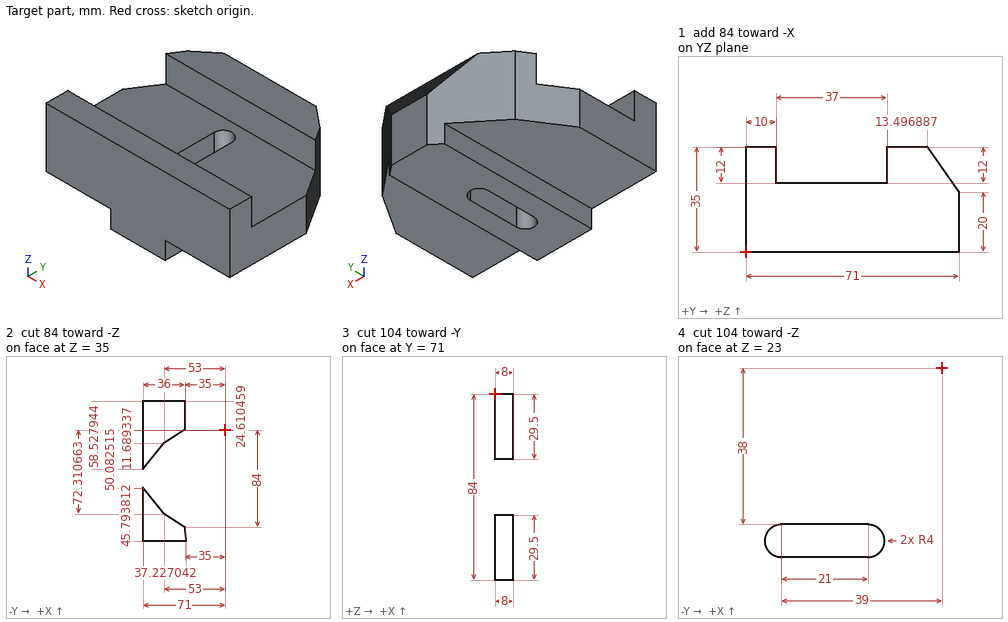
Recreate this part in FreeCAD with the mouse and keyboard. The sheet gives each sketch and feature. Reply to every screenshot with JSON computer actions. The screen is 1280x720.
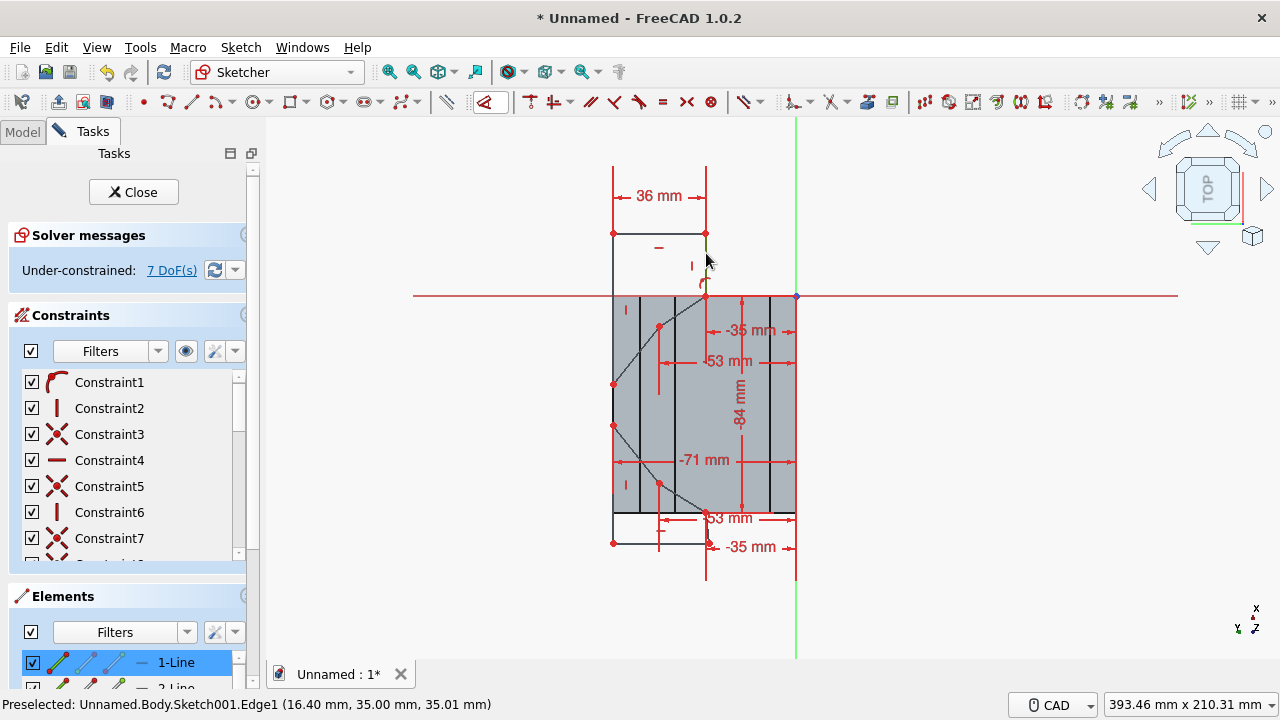
{"action": "left_click", "coordinate": [502, 102]}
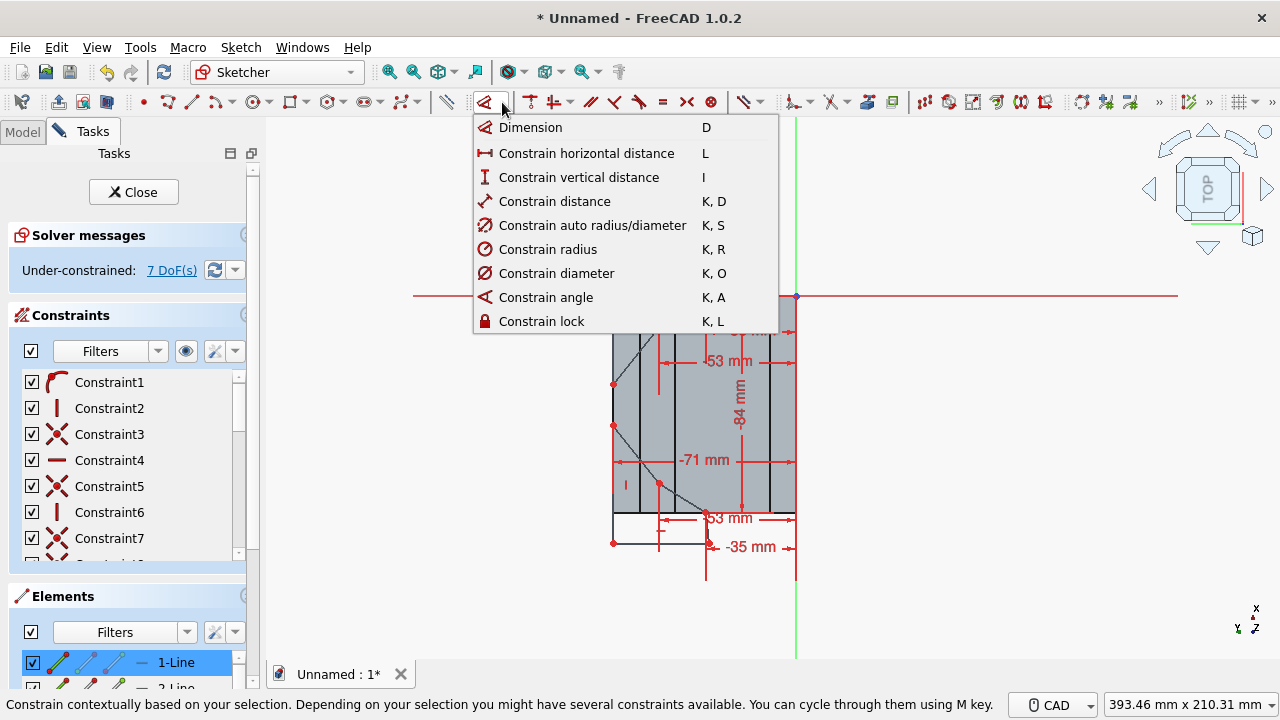
{"action": "left_click", "coordinate": [626, 177]}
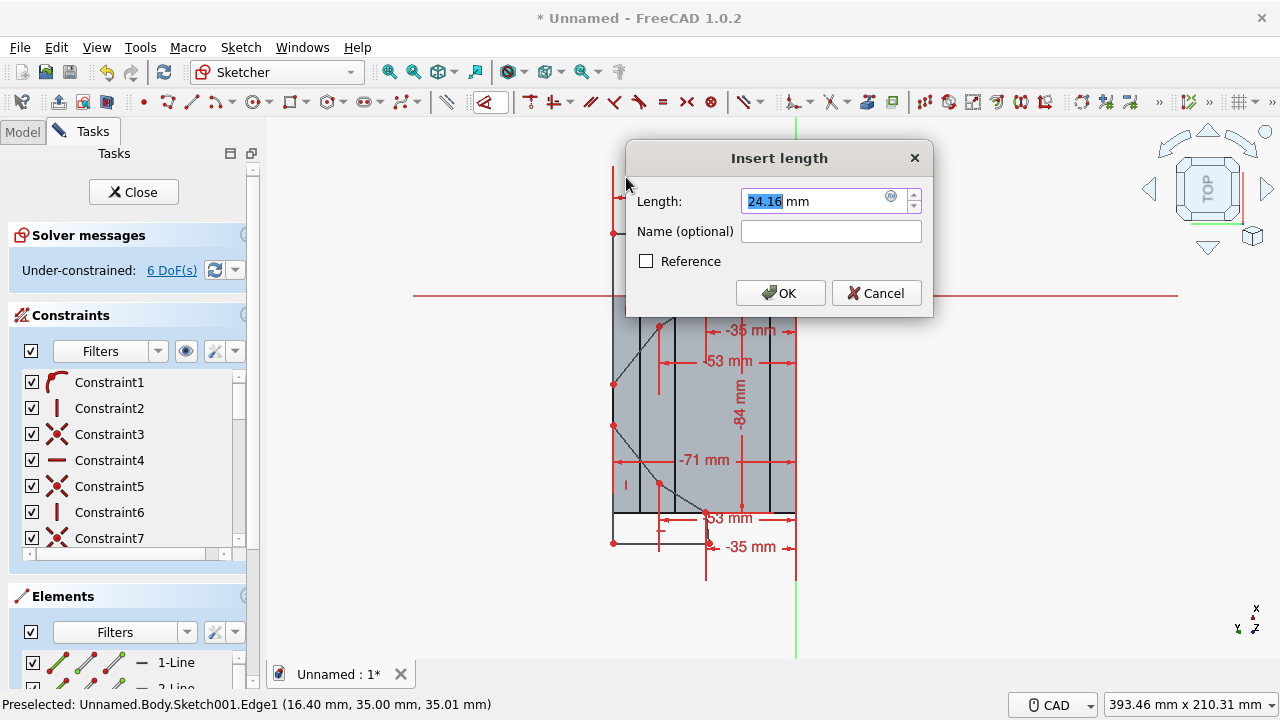
{"action": "type", "text": "24.610459"}
{"action": "key", "text": "Return"}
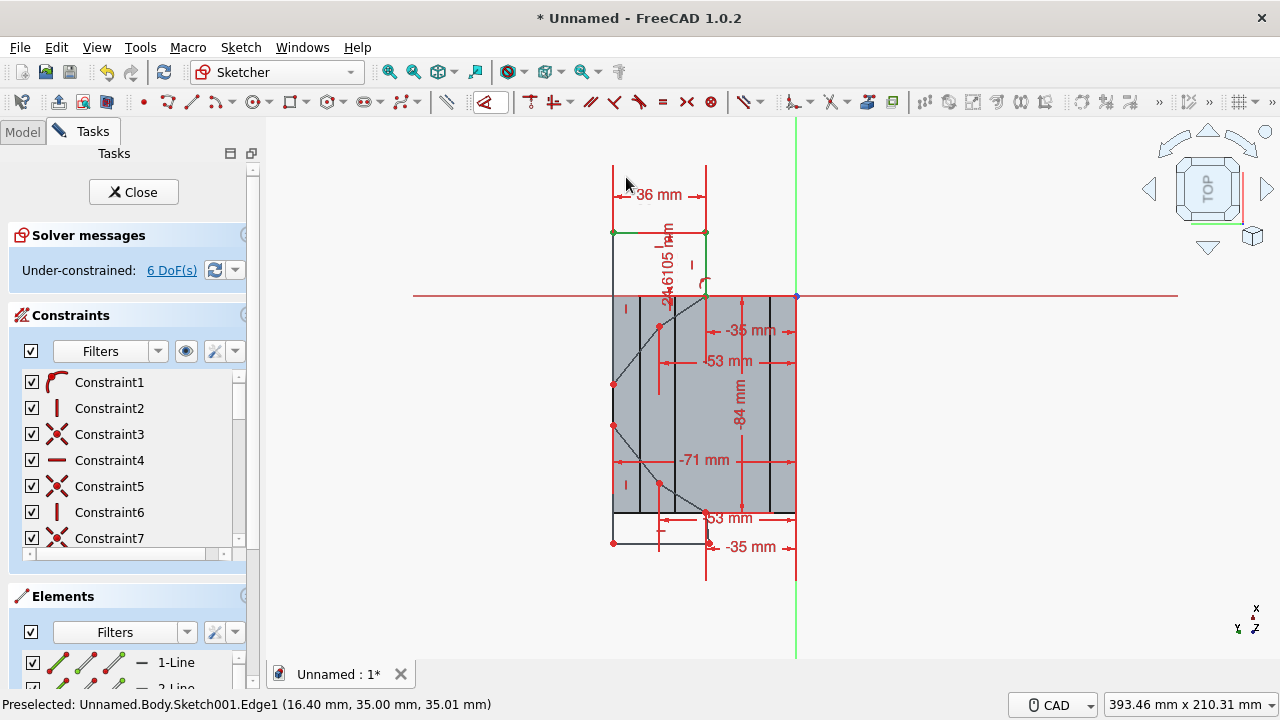
{"action": "left_click", "coordinate": [613, 278]}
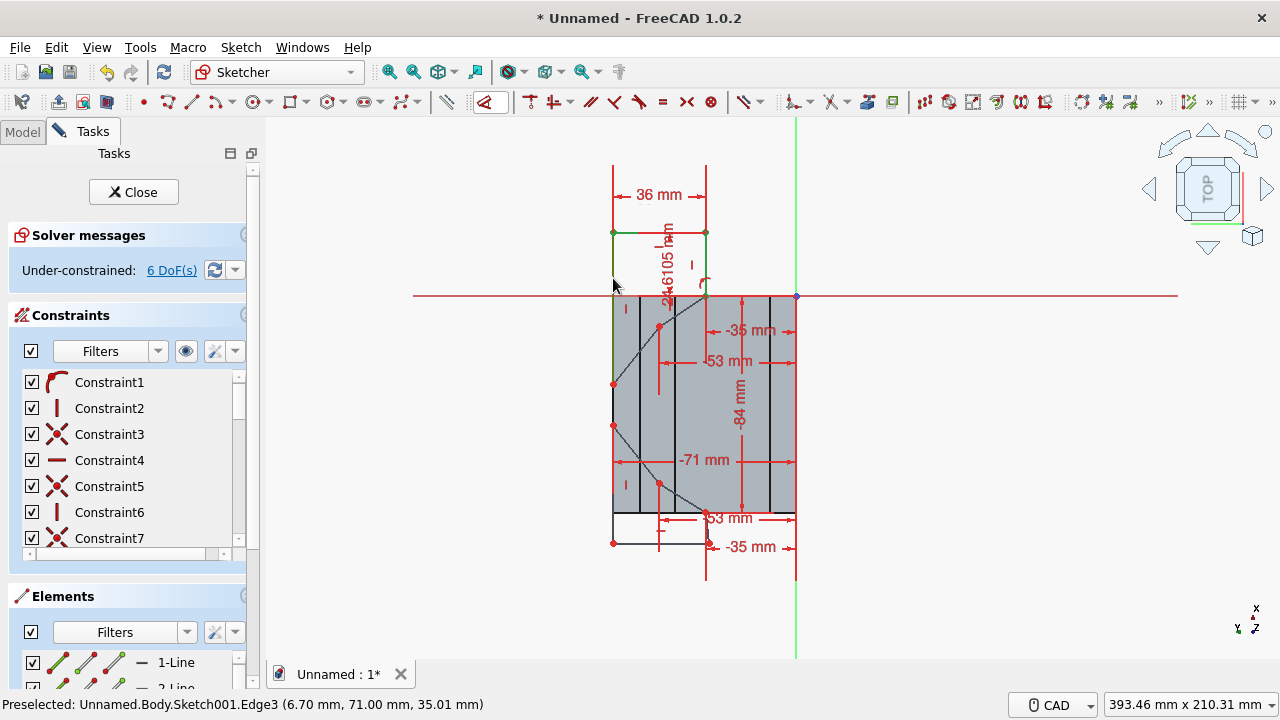
{"action": "left_click", "coordinate": [502, 102]}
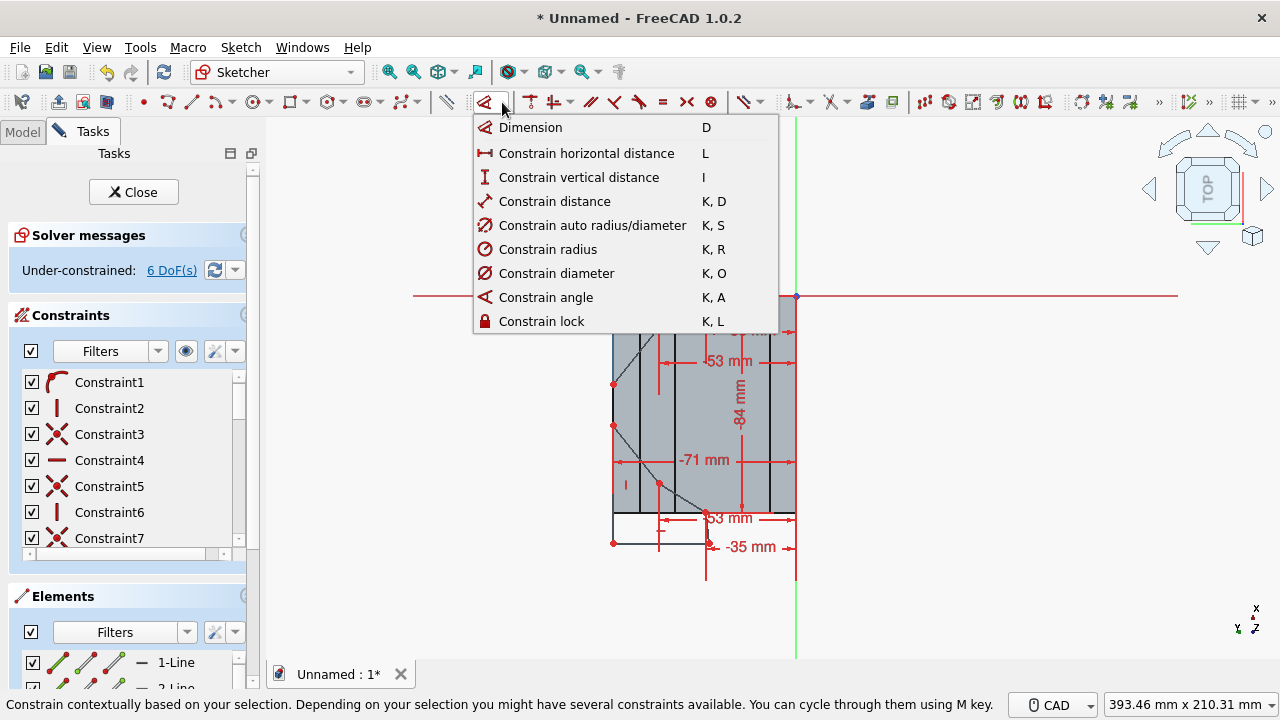
{"action": "left_click", "coordinate": [626, 177]}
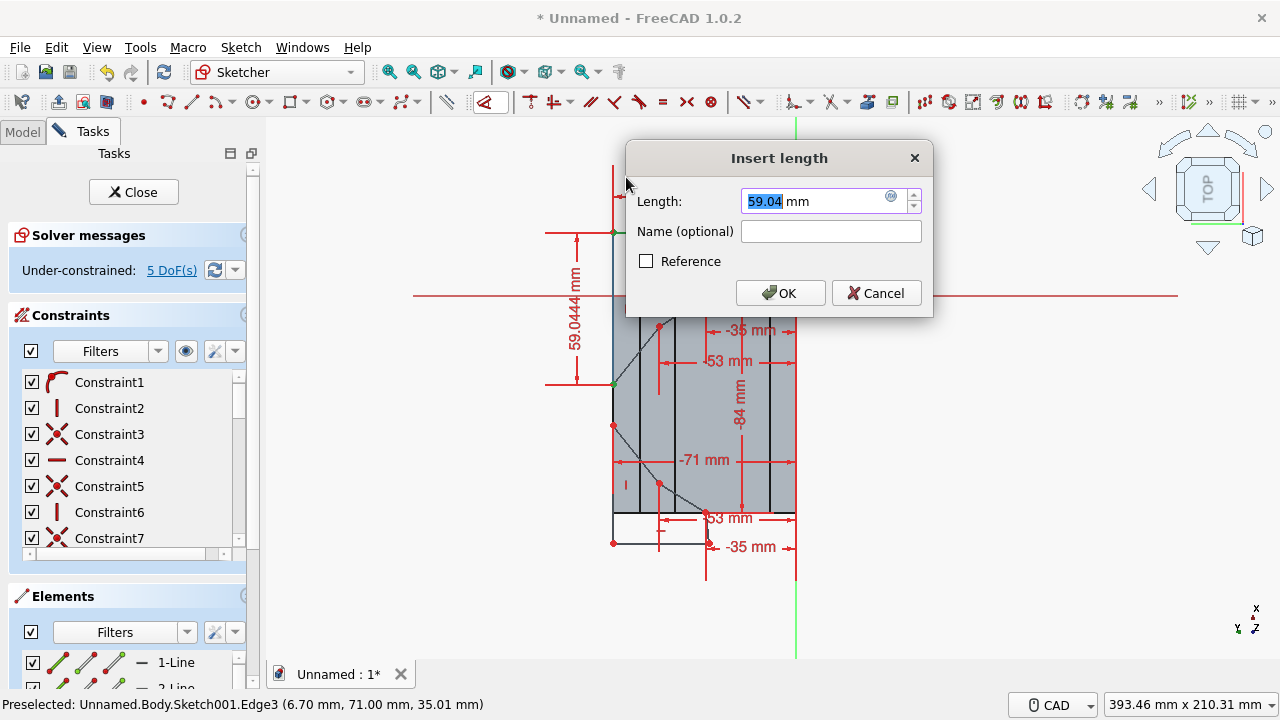
{"action": "type", "text": "58.527944"}
{"action": "key", "text": "Return"}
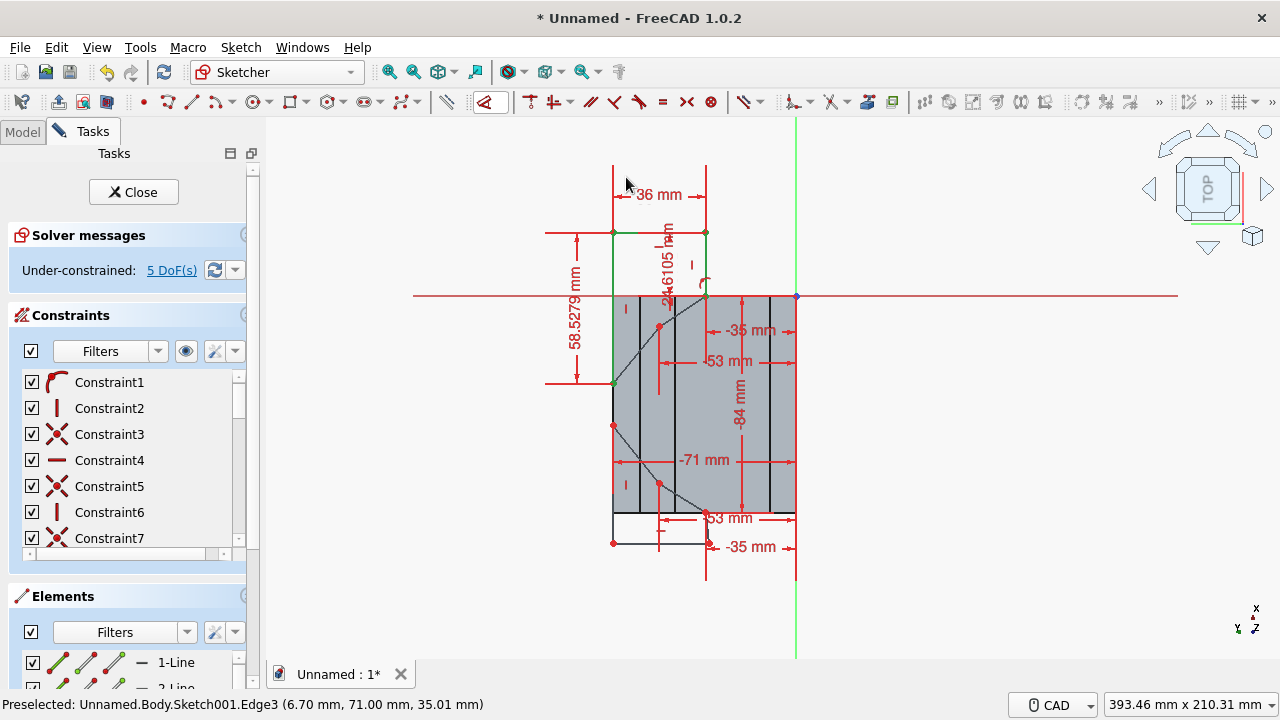
{"action": "left_click", "coordinate": [613, 461]}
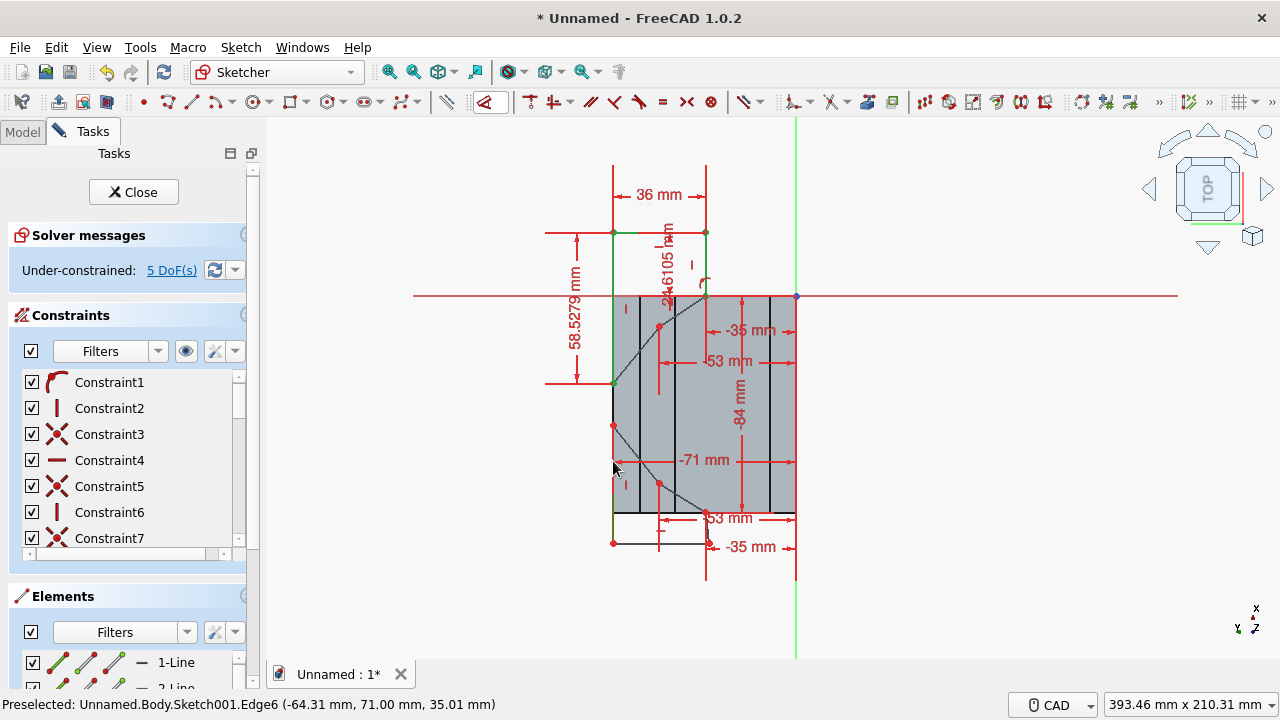
{"action": "left_click", "coordinate": [502, 102]}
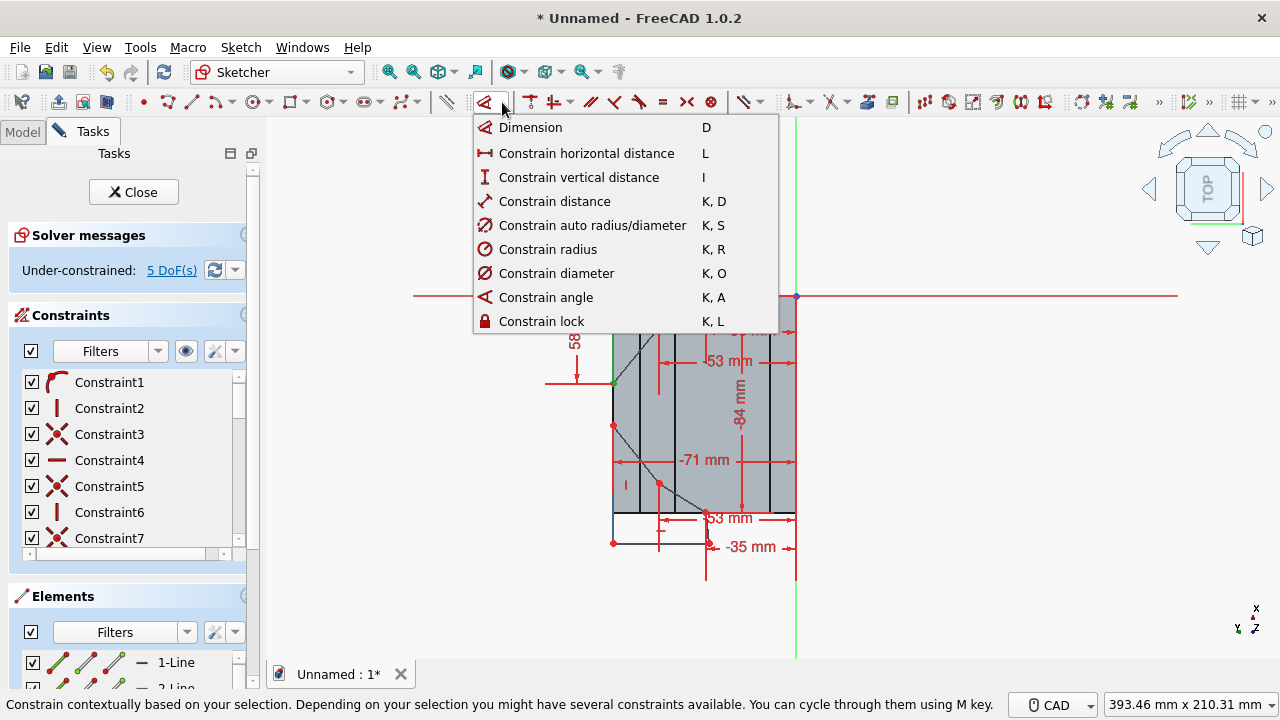
{"action": "left_click", "coordinate": [626, 177]}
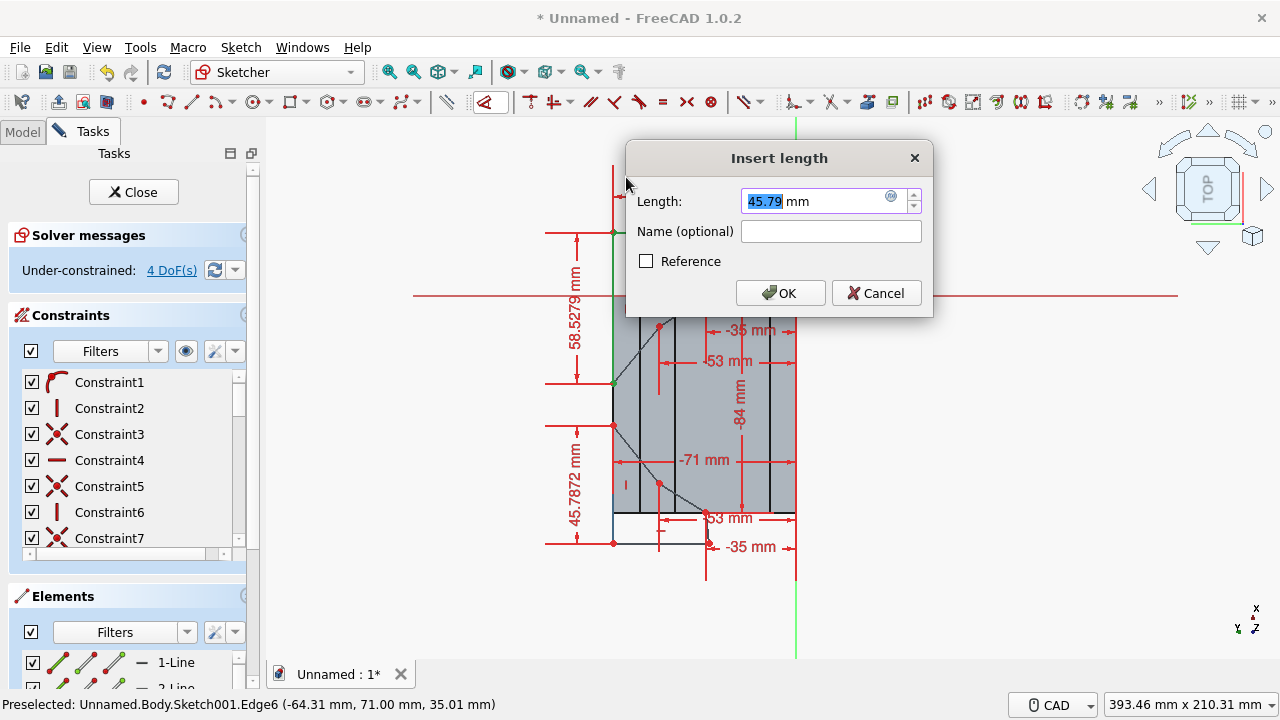
{"action": "type", "text": "45.793812"}
{"action": "key", "text": "Return"}